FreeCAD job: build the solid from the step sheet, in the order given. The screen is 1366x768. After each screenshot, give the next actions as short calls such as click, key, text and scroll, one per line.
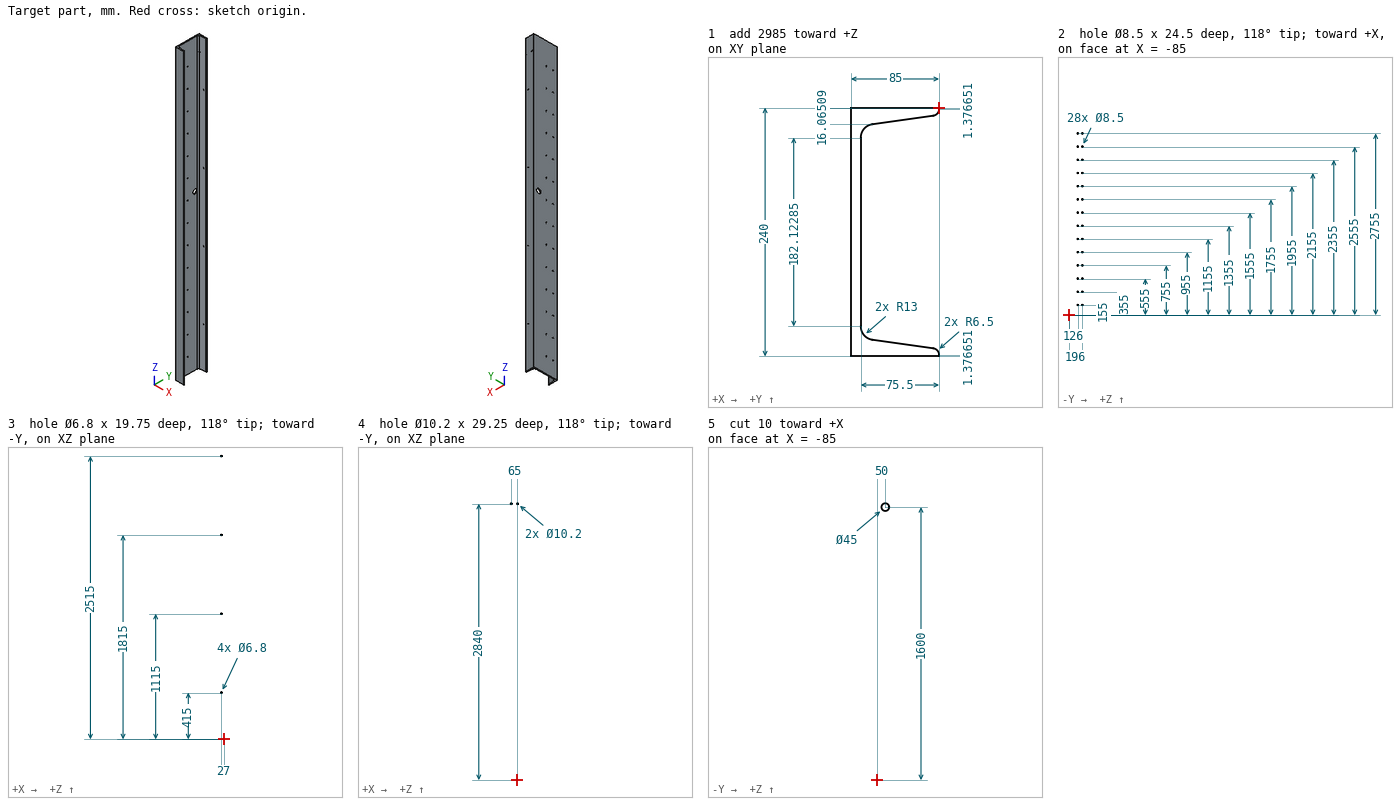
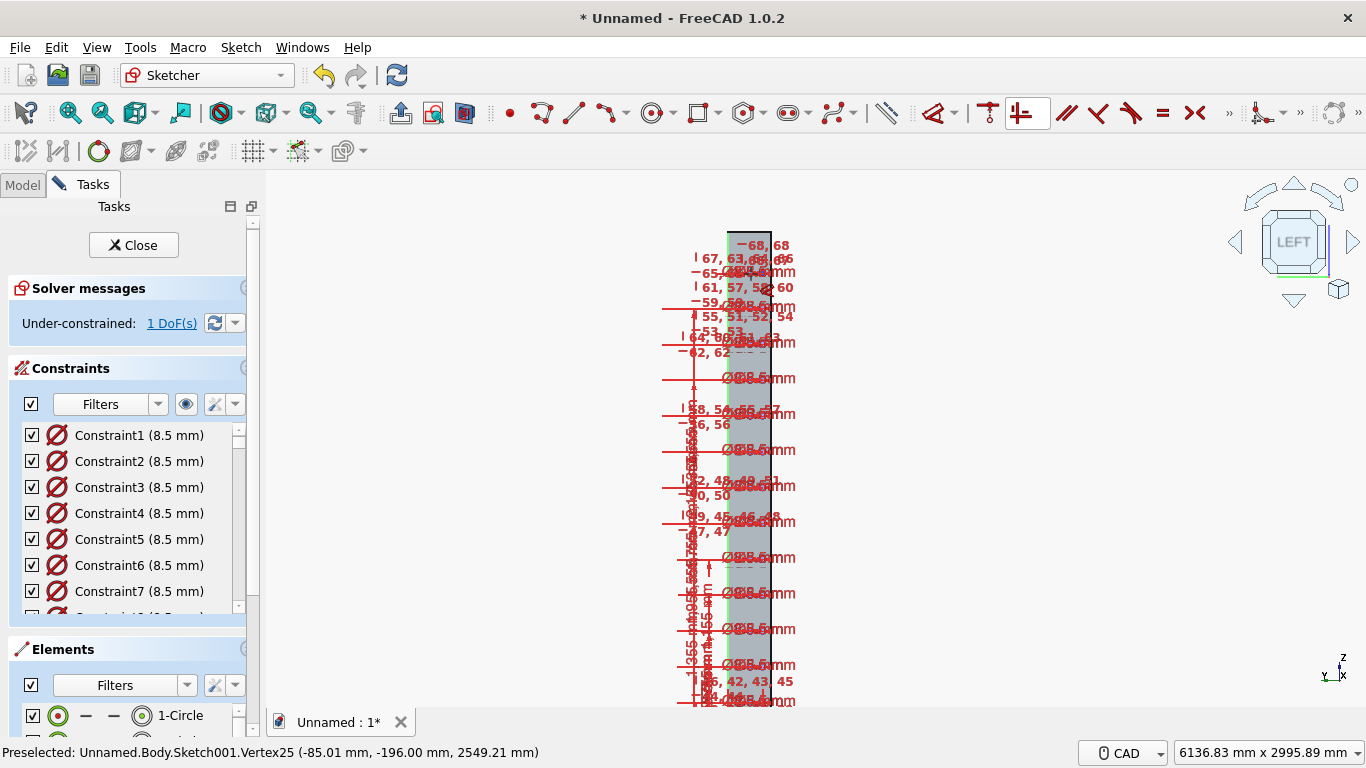
click(750, 274)
click(694, 383)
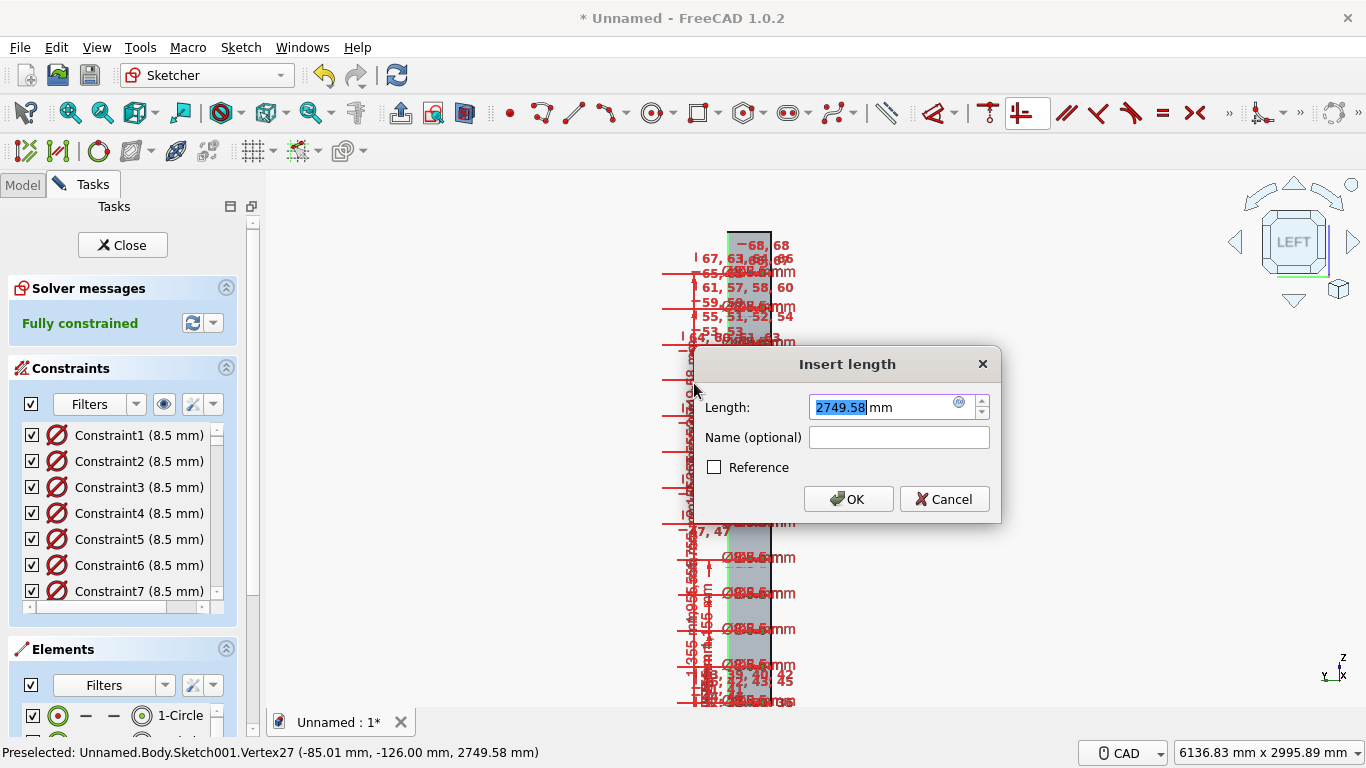
text(2755)
key(Return)
key(Escape)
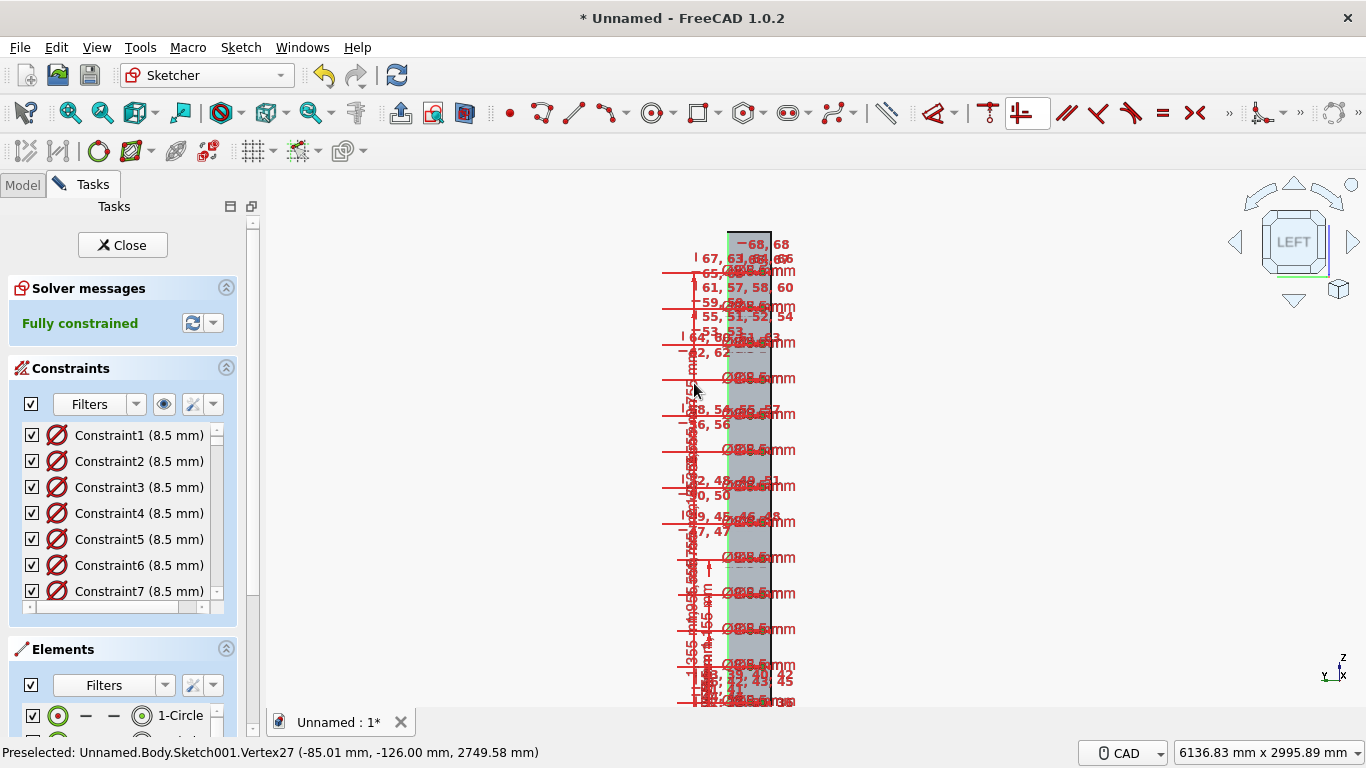
click(123, 245)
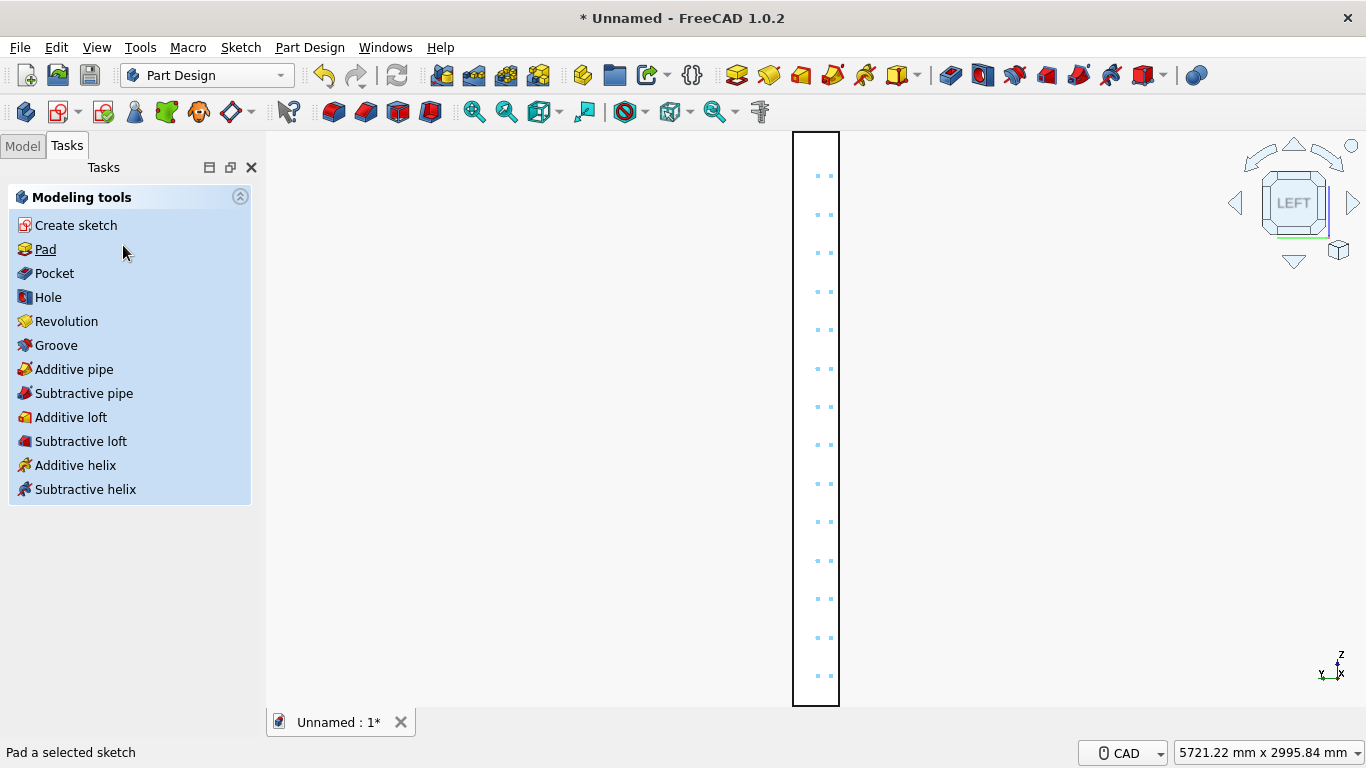
click(984, 76)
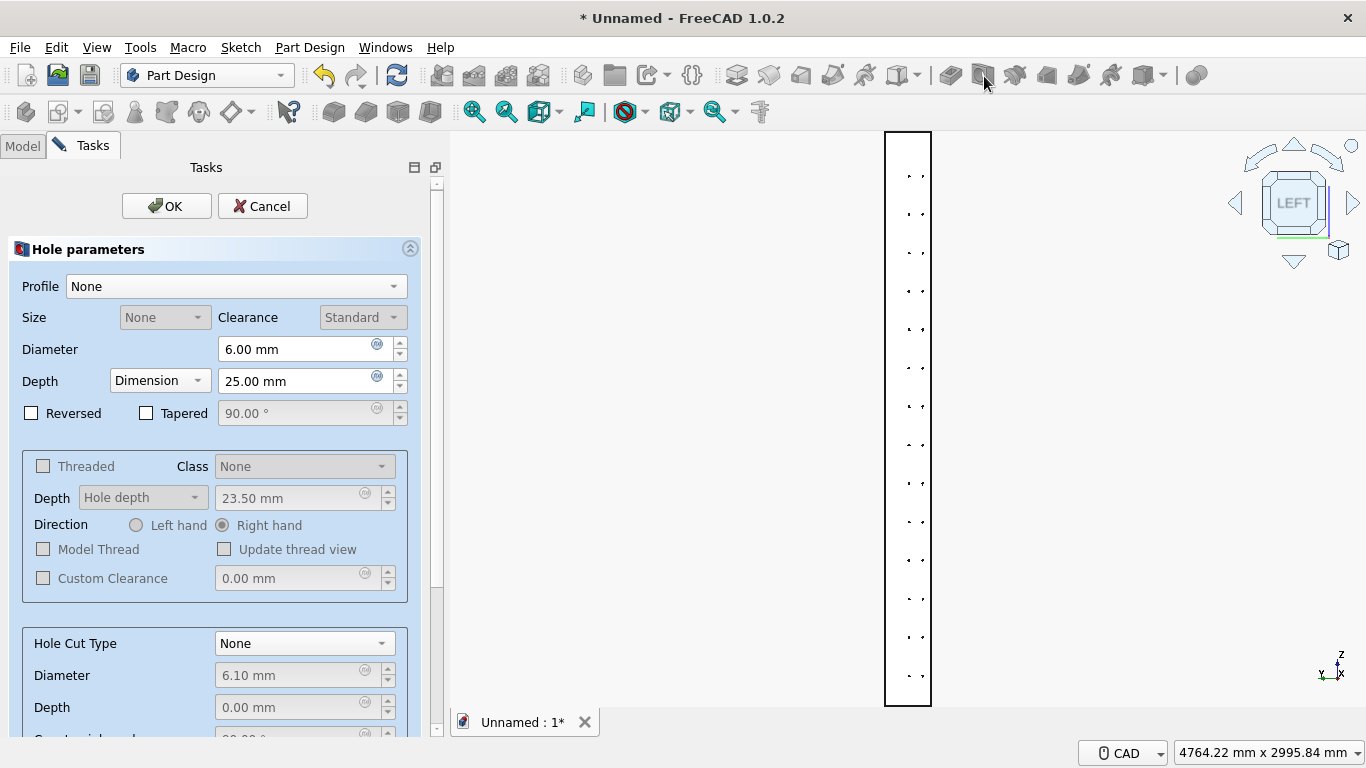
triple_click(305, 349)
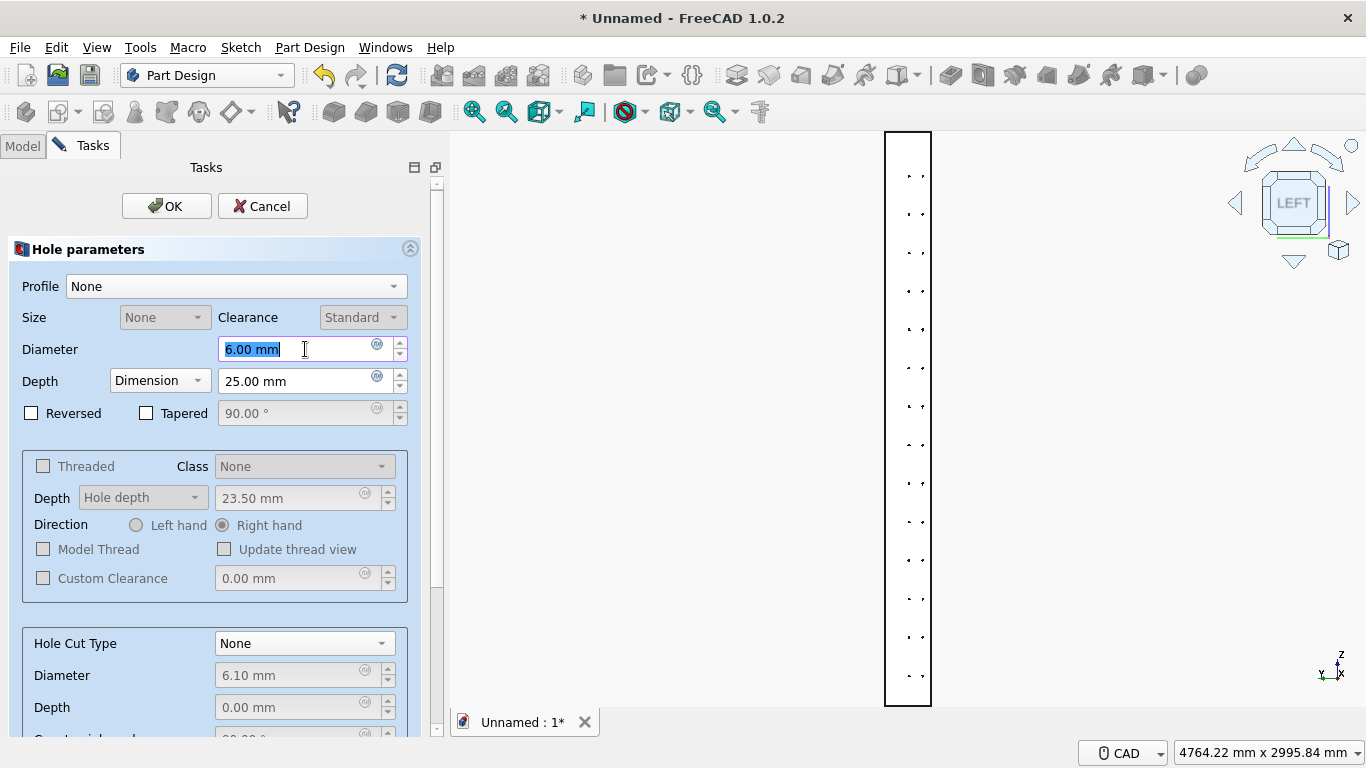
text(8.5)
key(Tab)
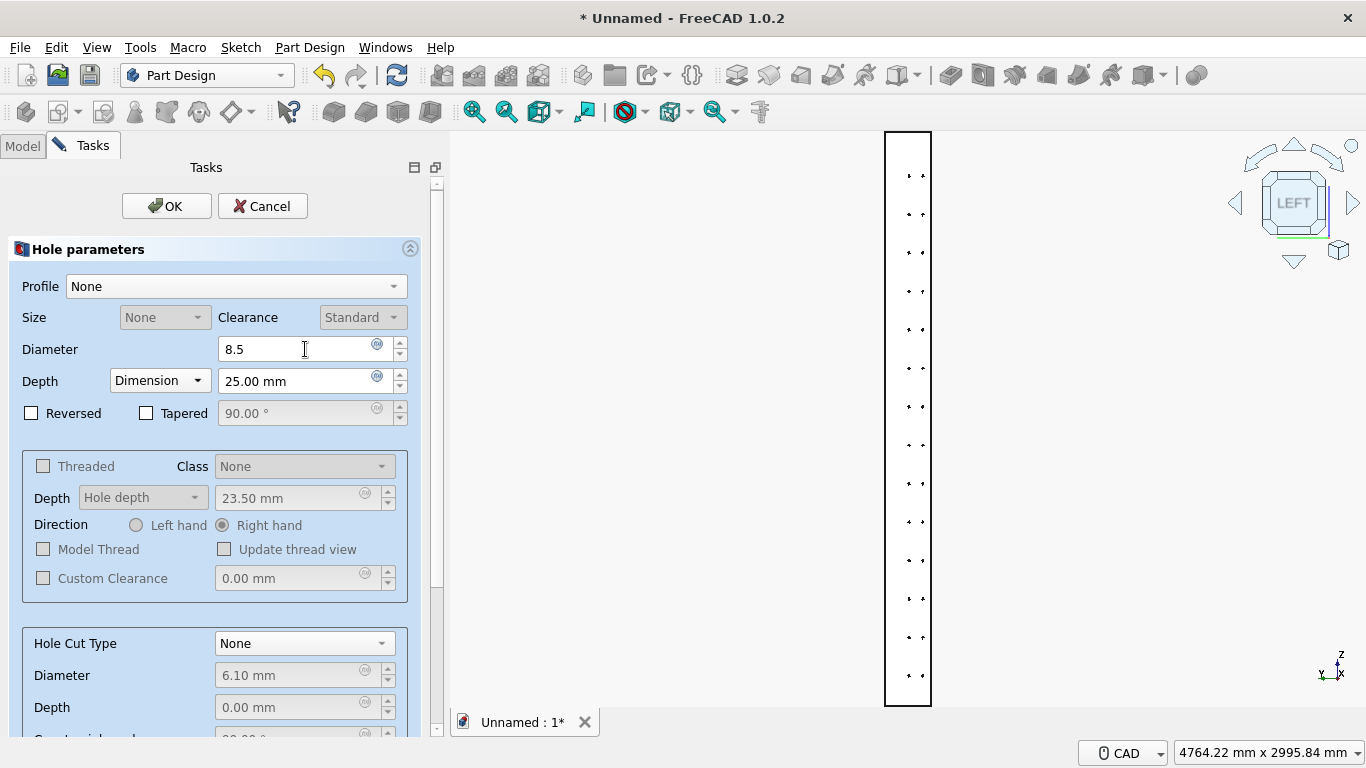
triple_click(305, 381)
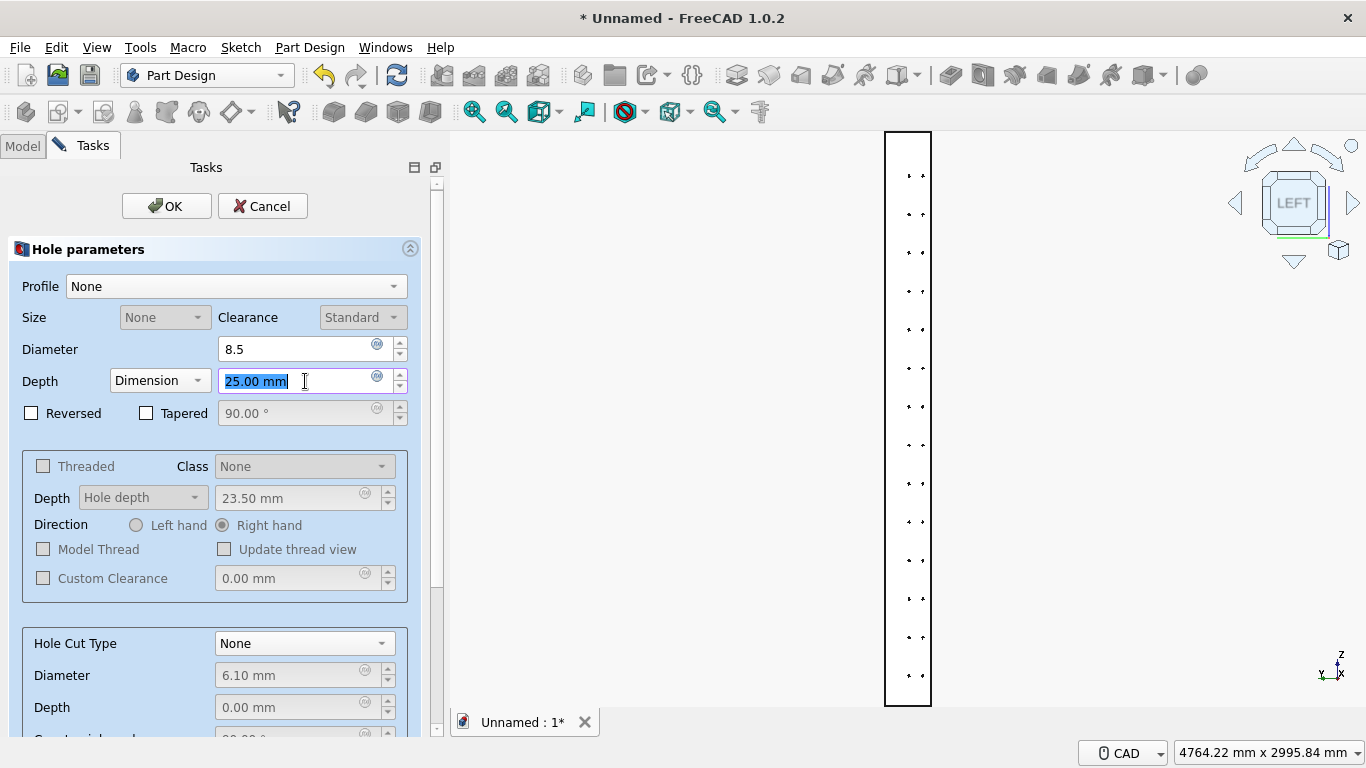
text(24.5)
key(Tab)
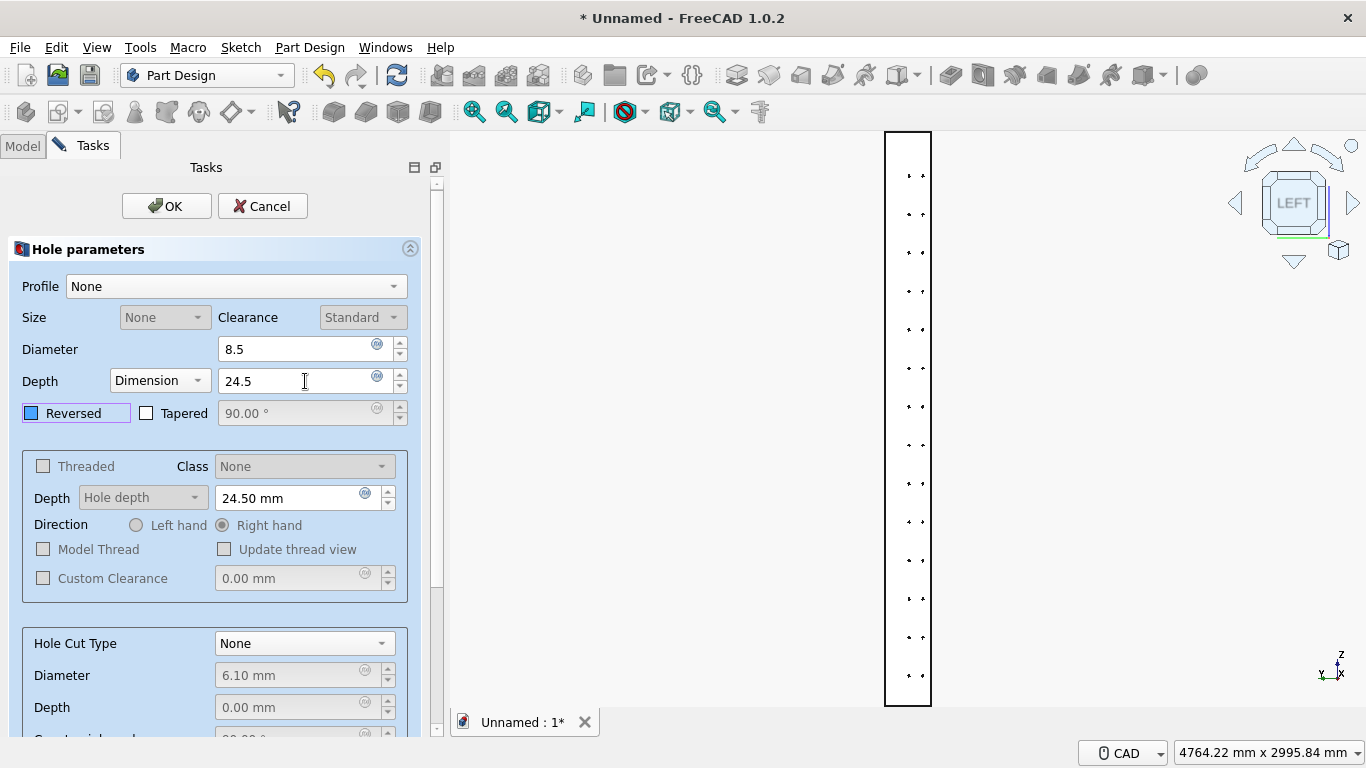
click(167, 206)